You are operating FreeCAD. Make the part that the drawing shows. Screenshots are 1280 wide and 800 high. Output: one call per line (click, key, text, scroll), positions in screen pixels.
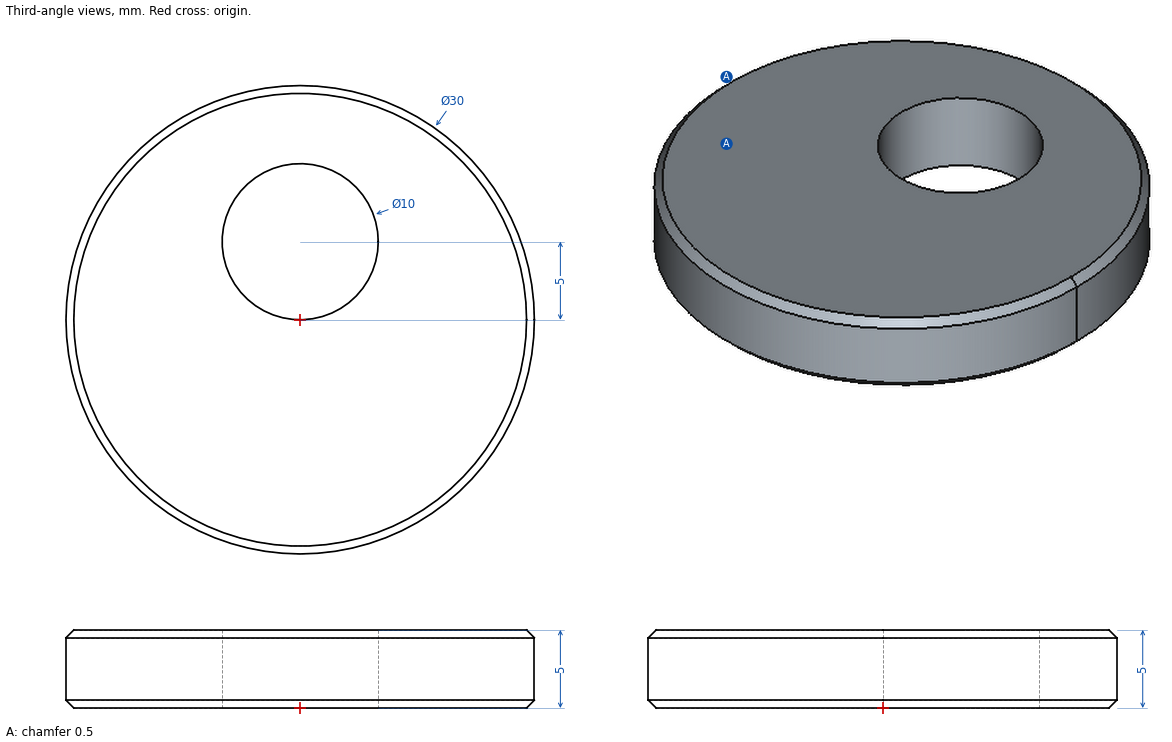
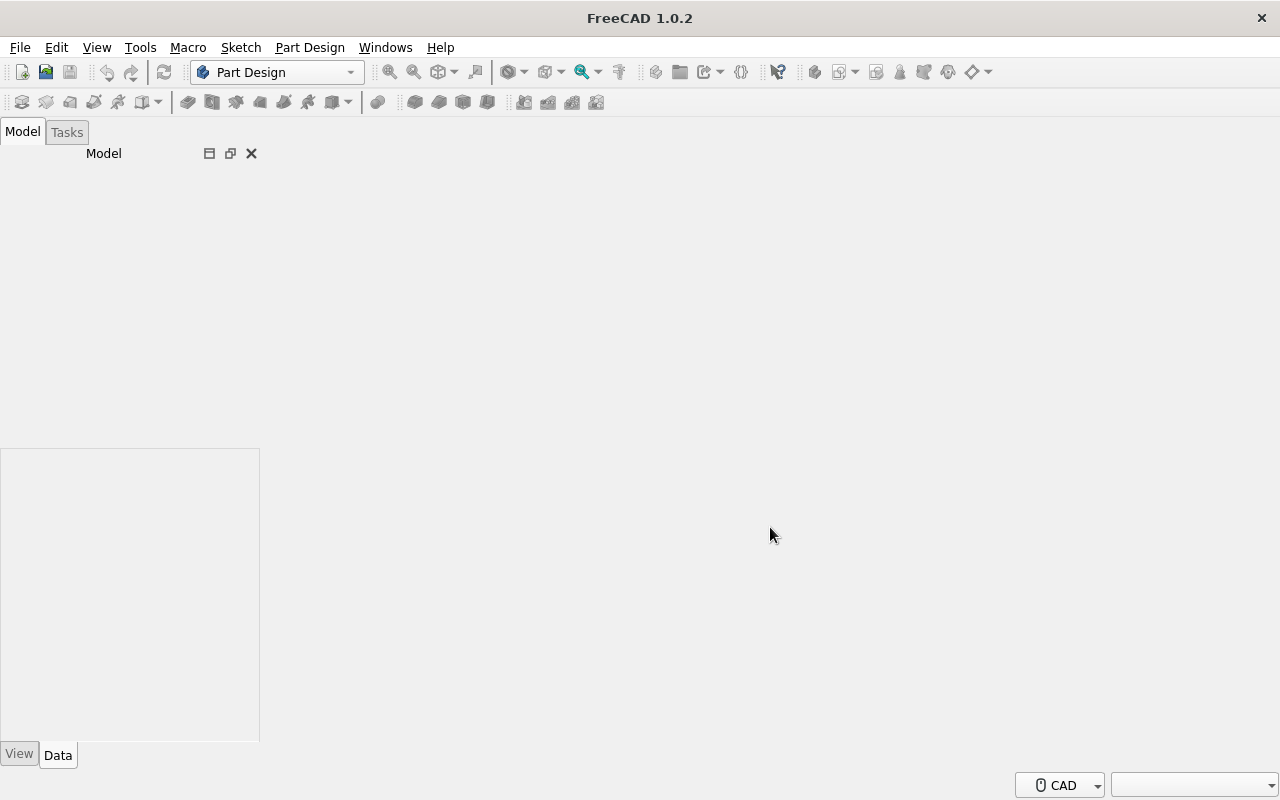
key(ctrl+n)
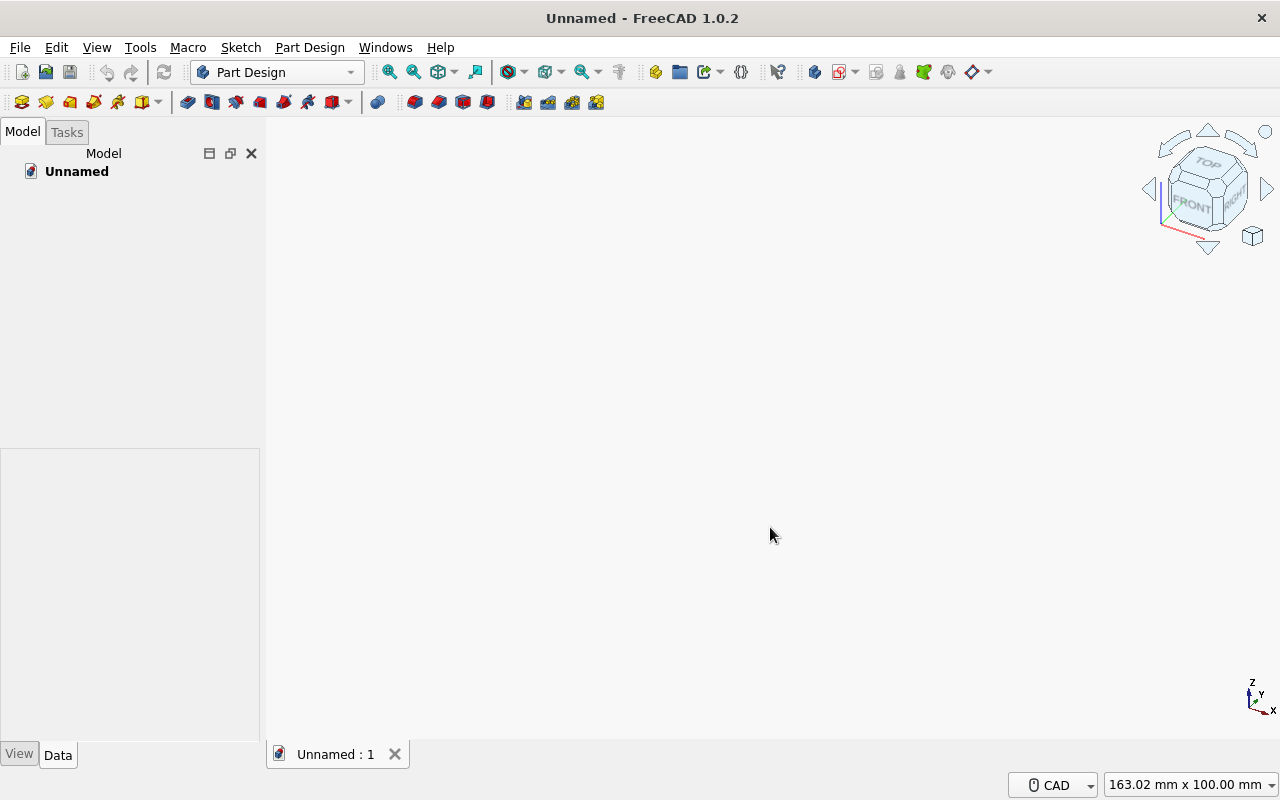
click(840, 72)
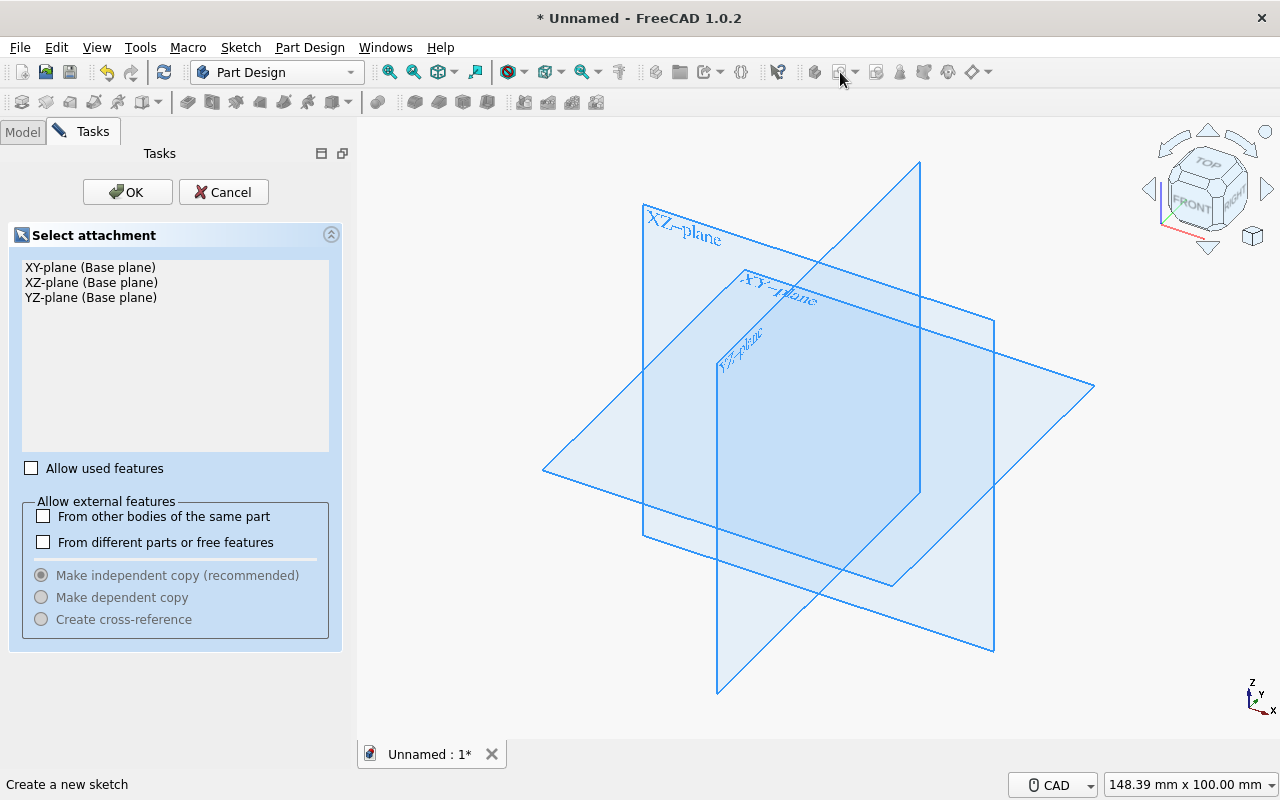
click(82, 268)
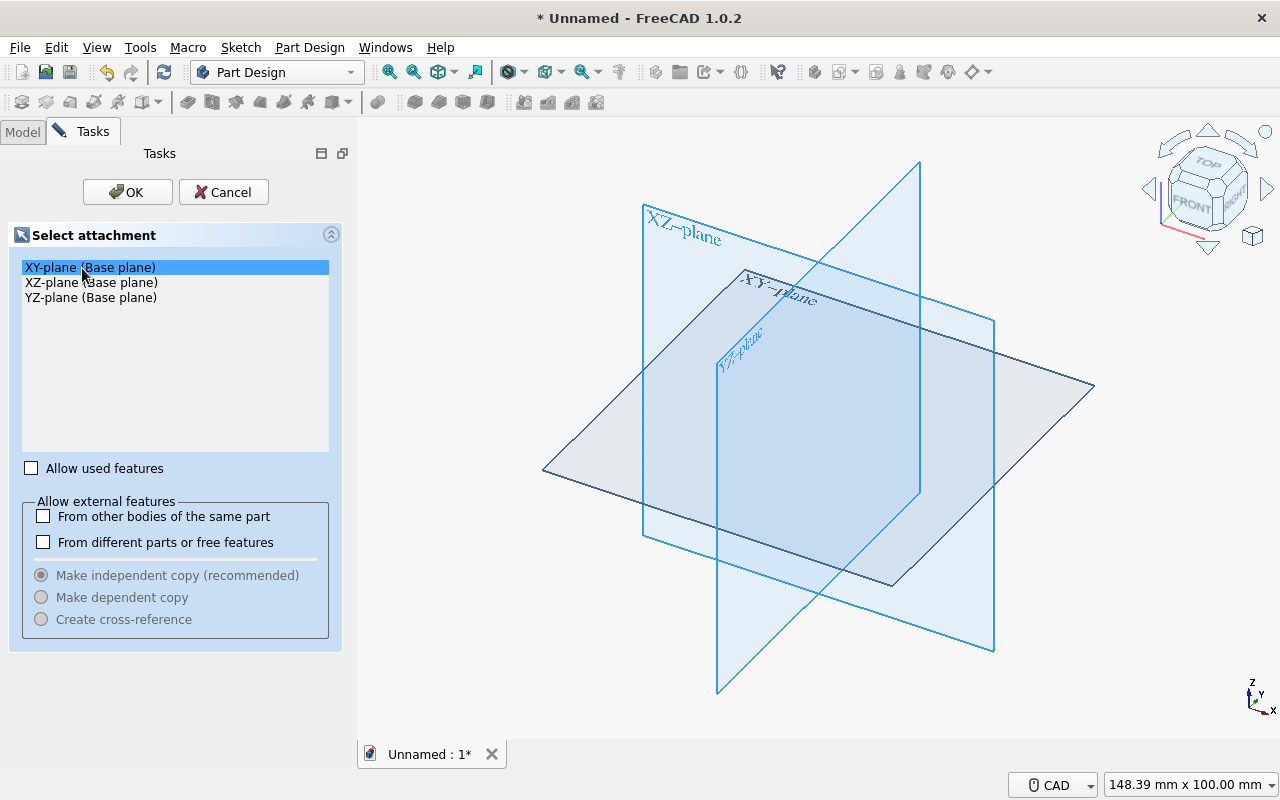
click(128, 192)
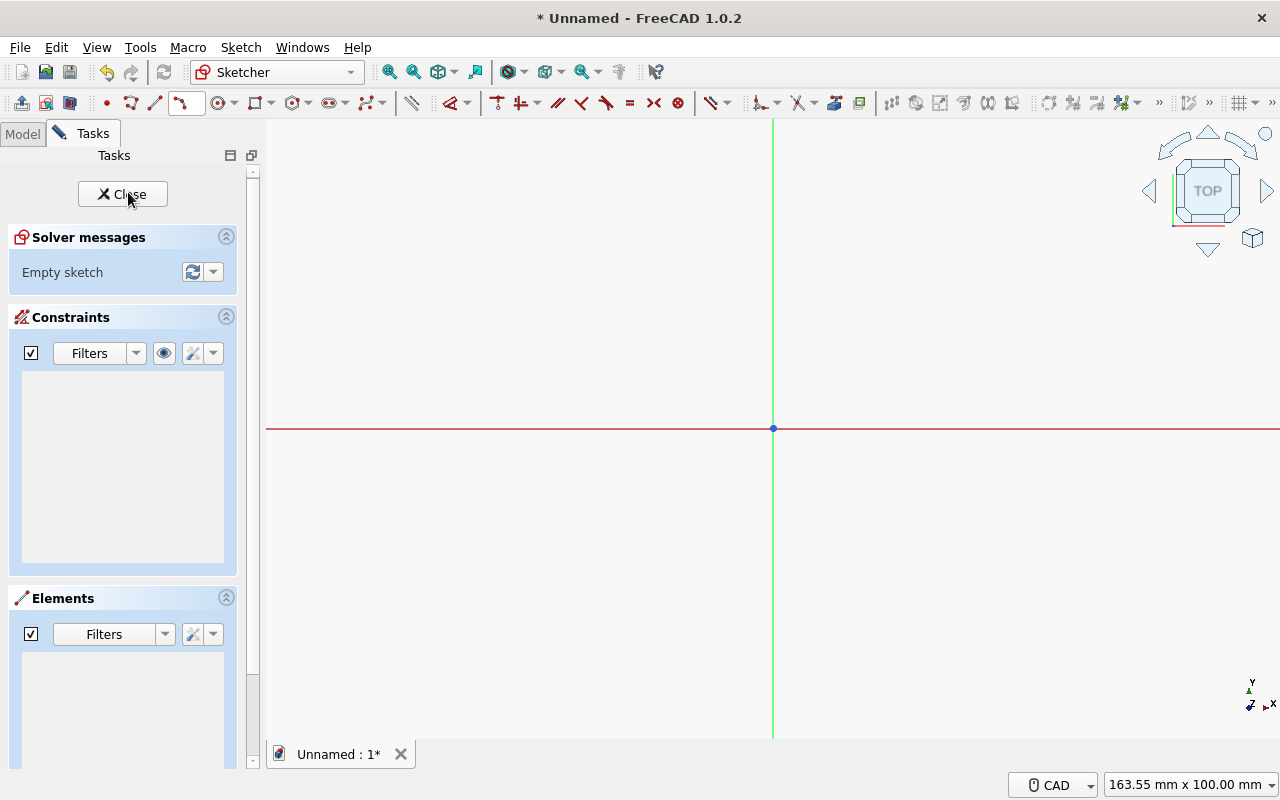
scroll(829, 429, up, 4)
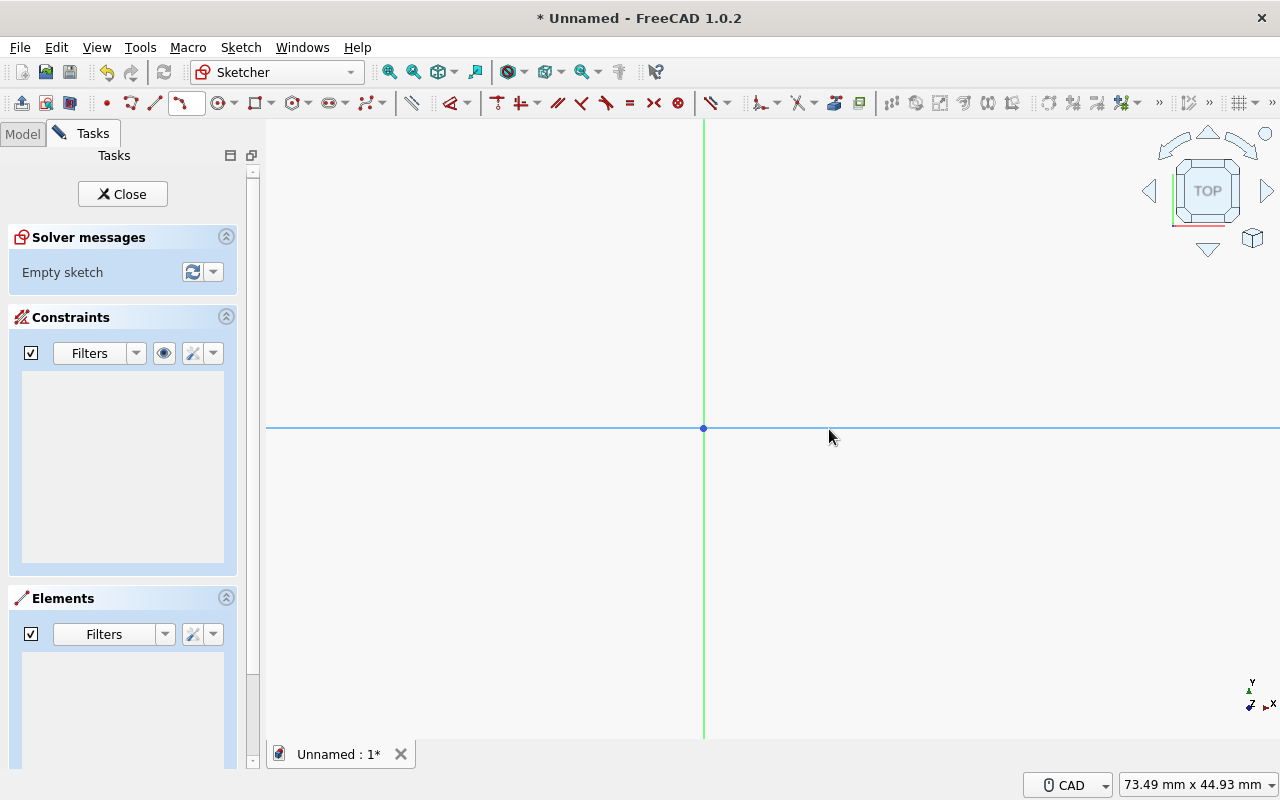
key(g)
key(c)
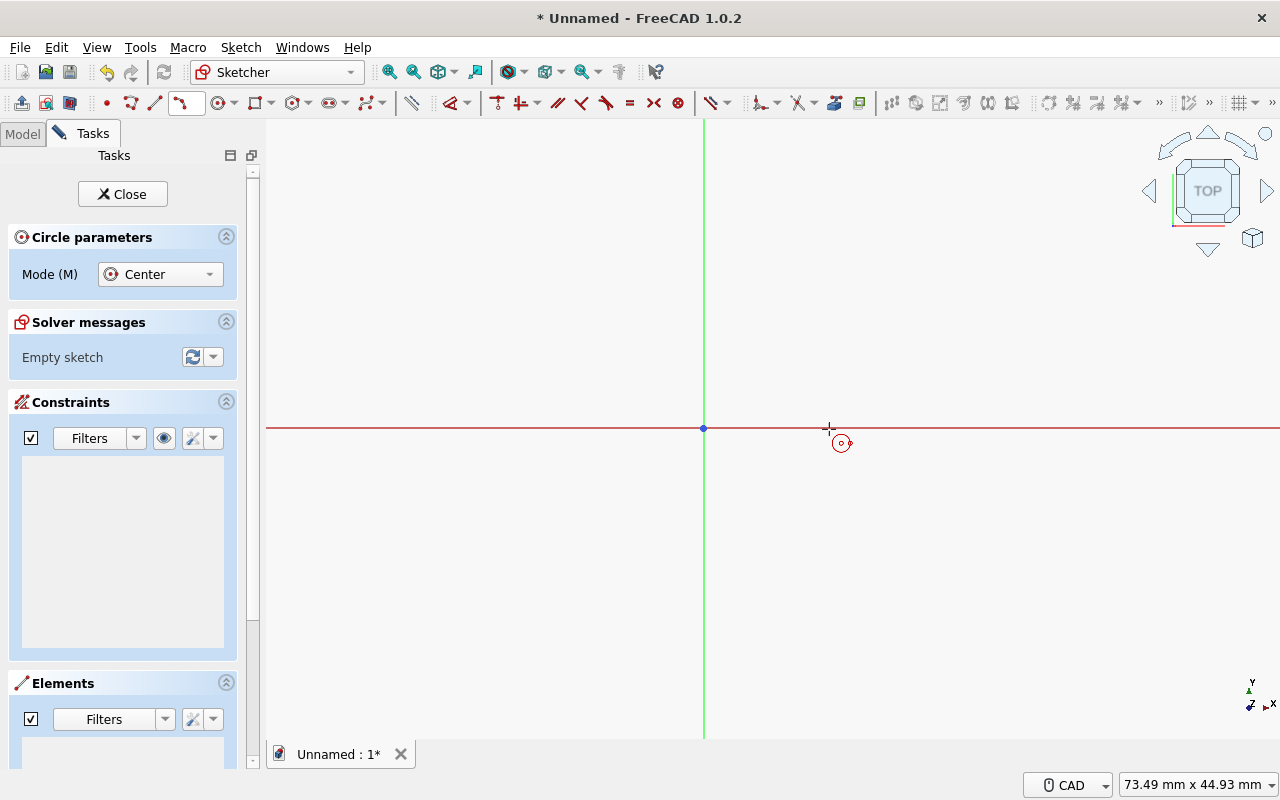
click(704, 428)
click(850, 282)
key(Escape)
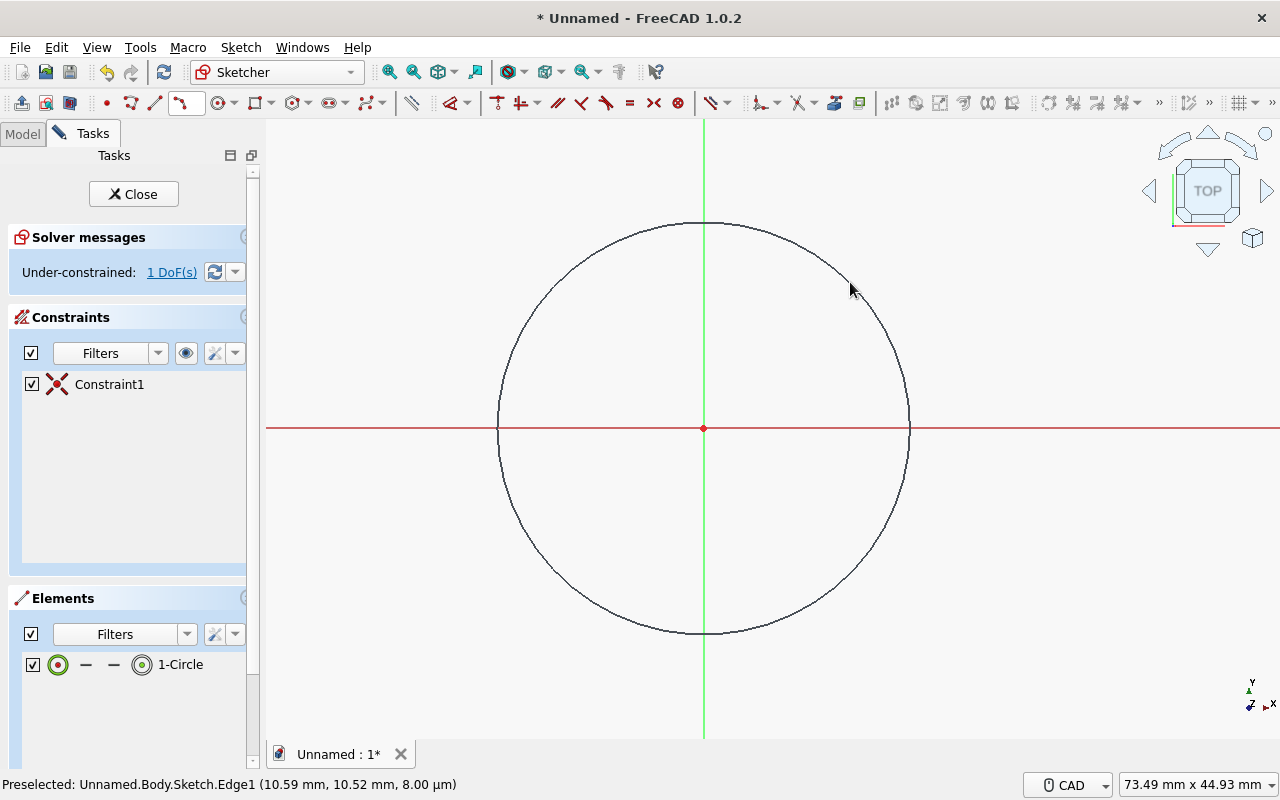
key(d)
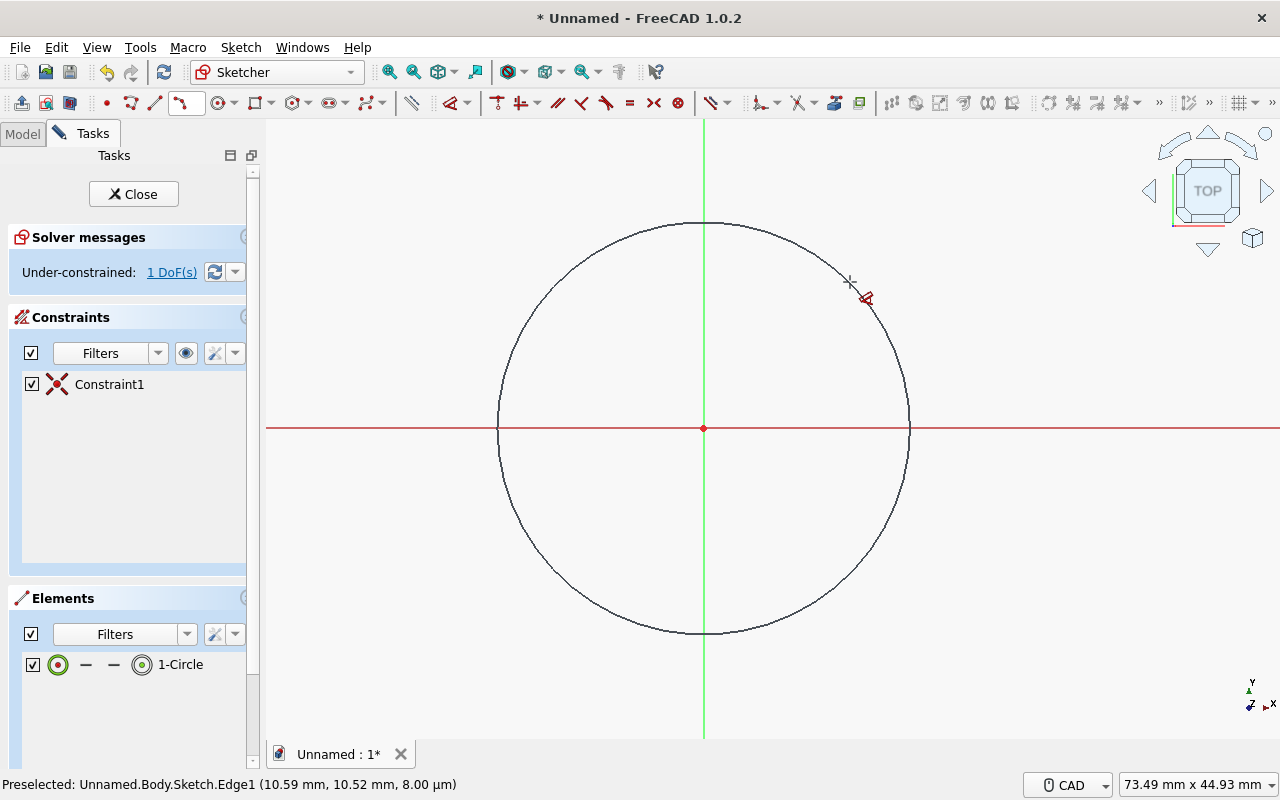
click(849, 282)
click(872, 259)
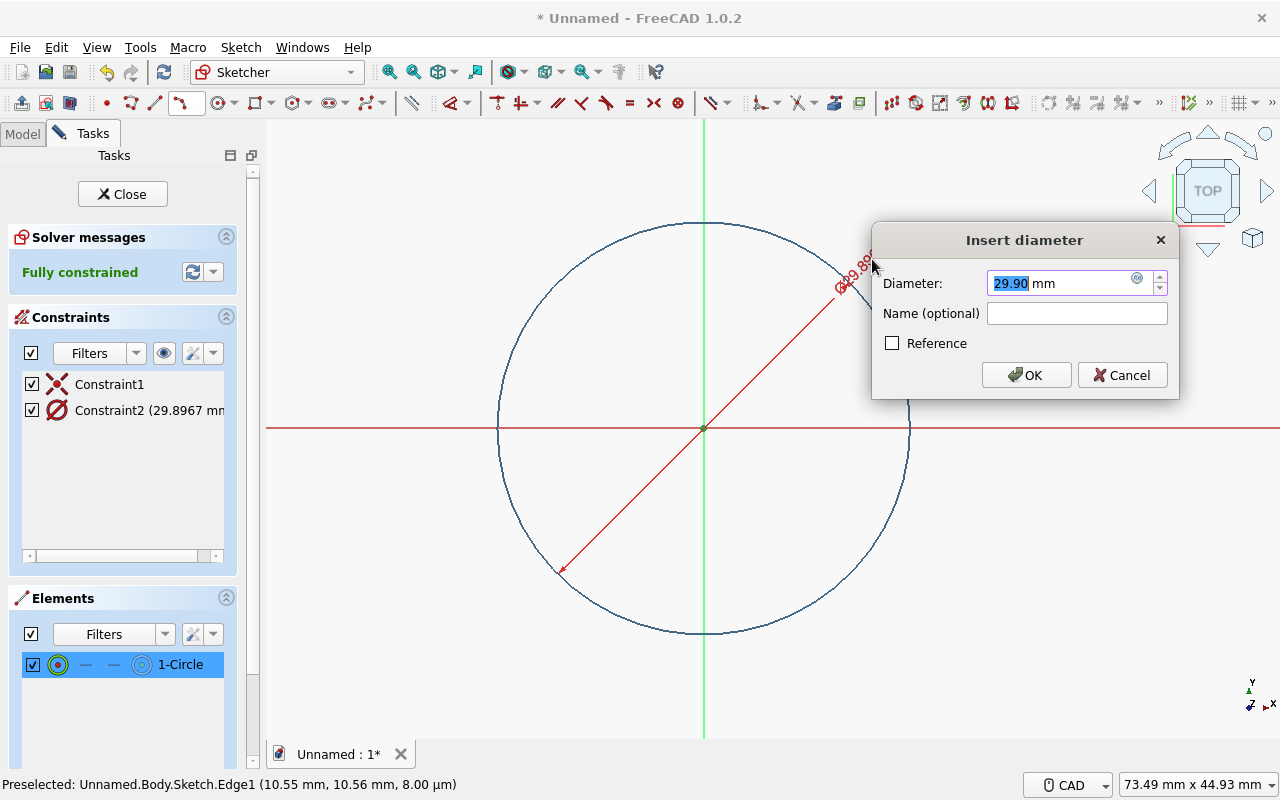
text(30)
key(Return)
key(Escape)